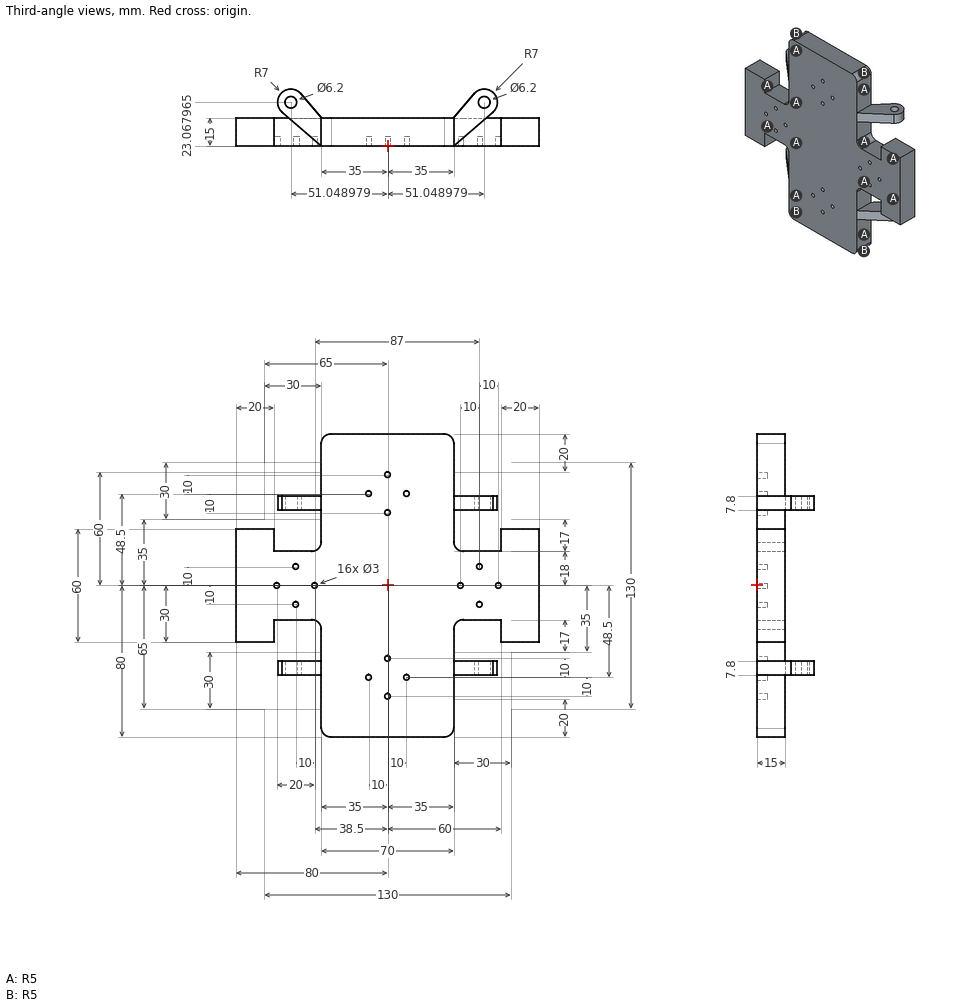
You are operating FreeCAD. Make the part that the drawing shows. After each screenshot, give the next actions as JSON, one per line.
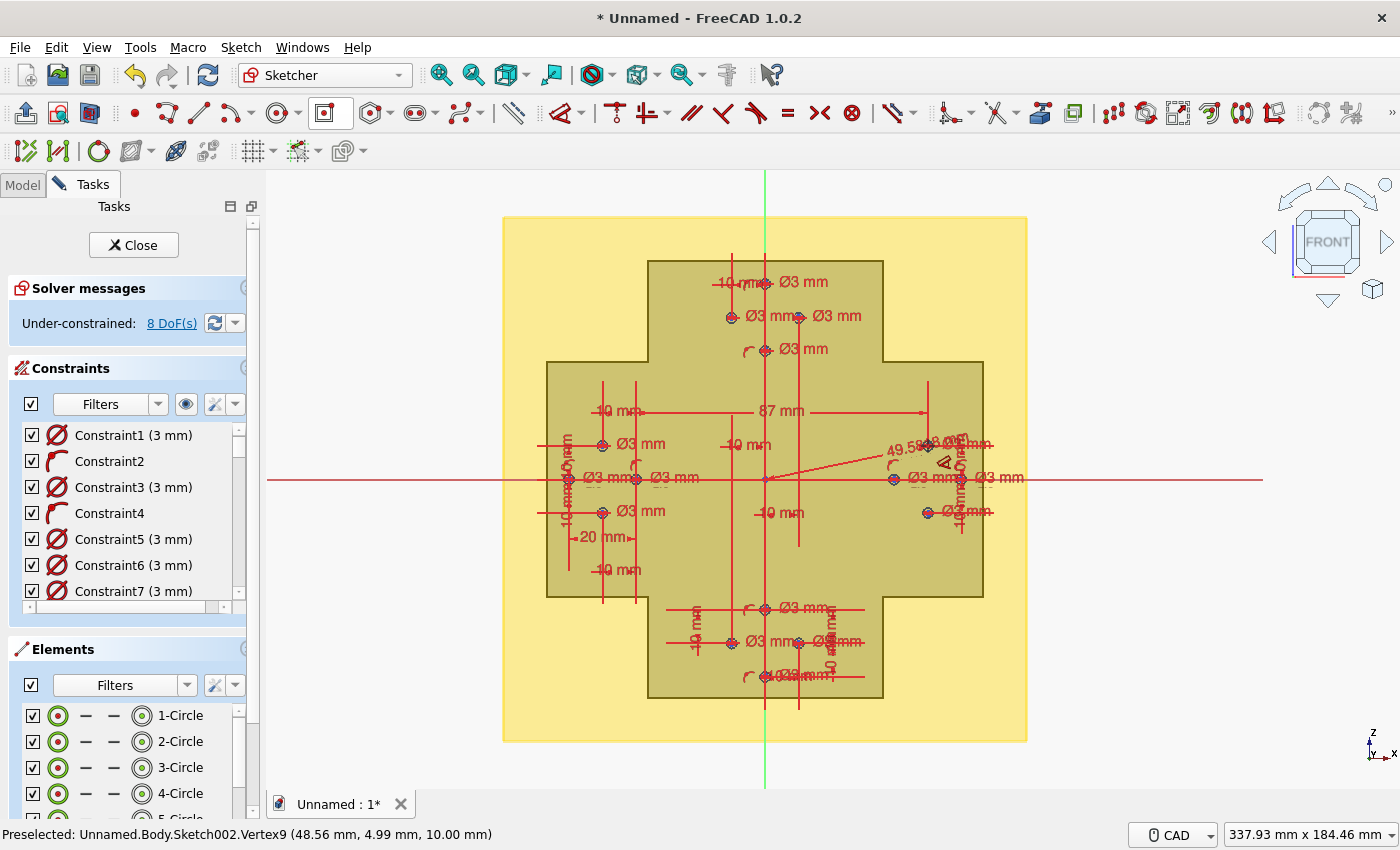
{"action": "left_click", "coordinate": [894, 480]}
{"action": "left_click", "coordinate": [911, 412]}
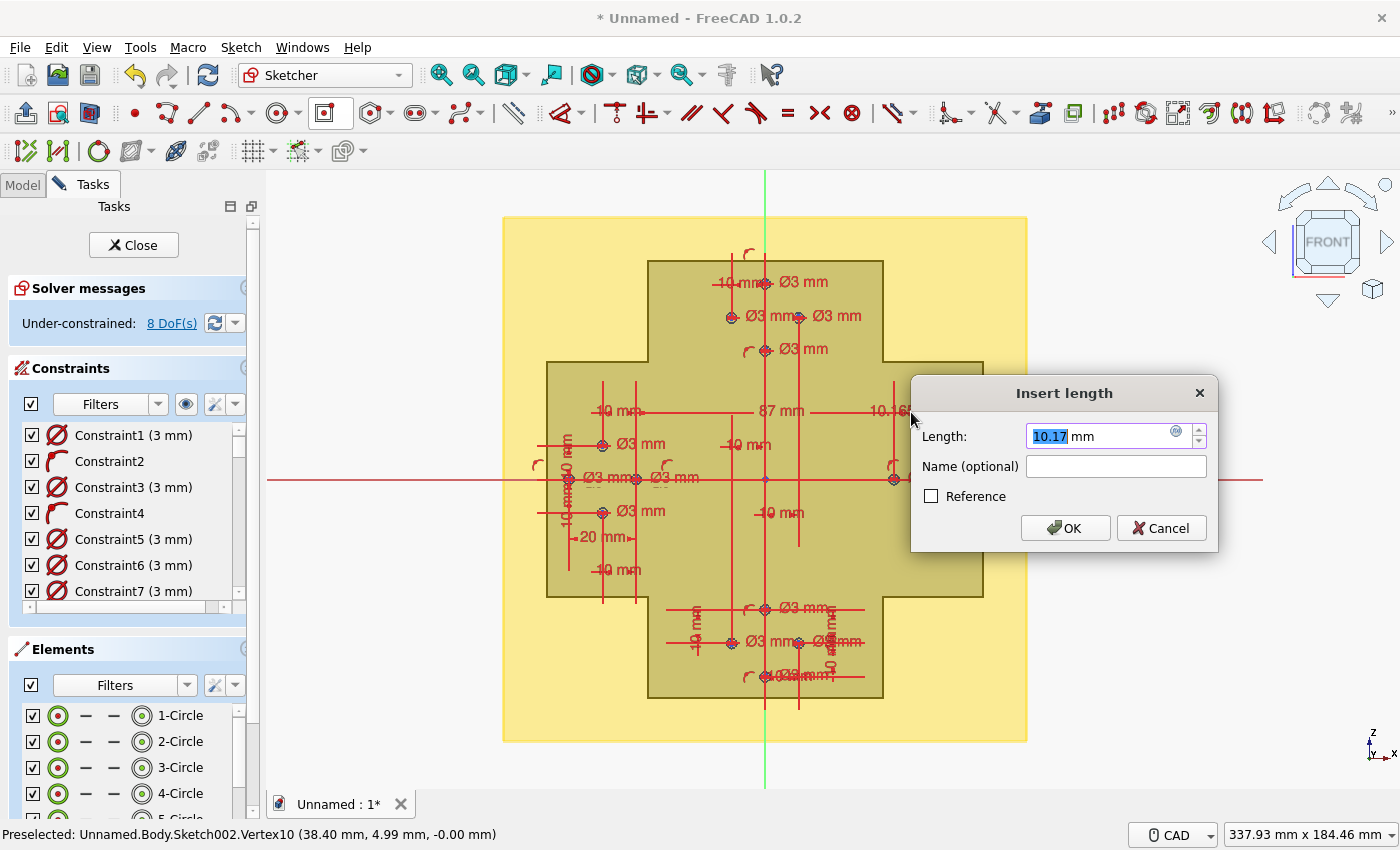
{"action": "type", "text": "10"}
{"action": "key", "text": "Return"}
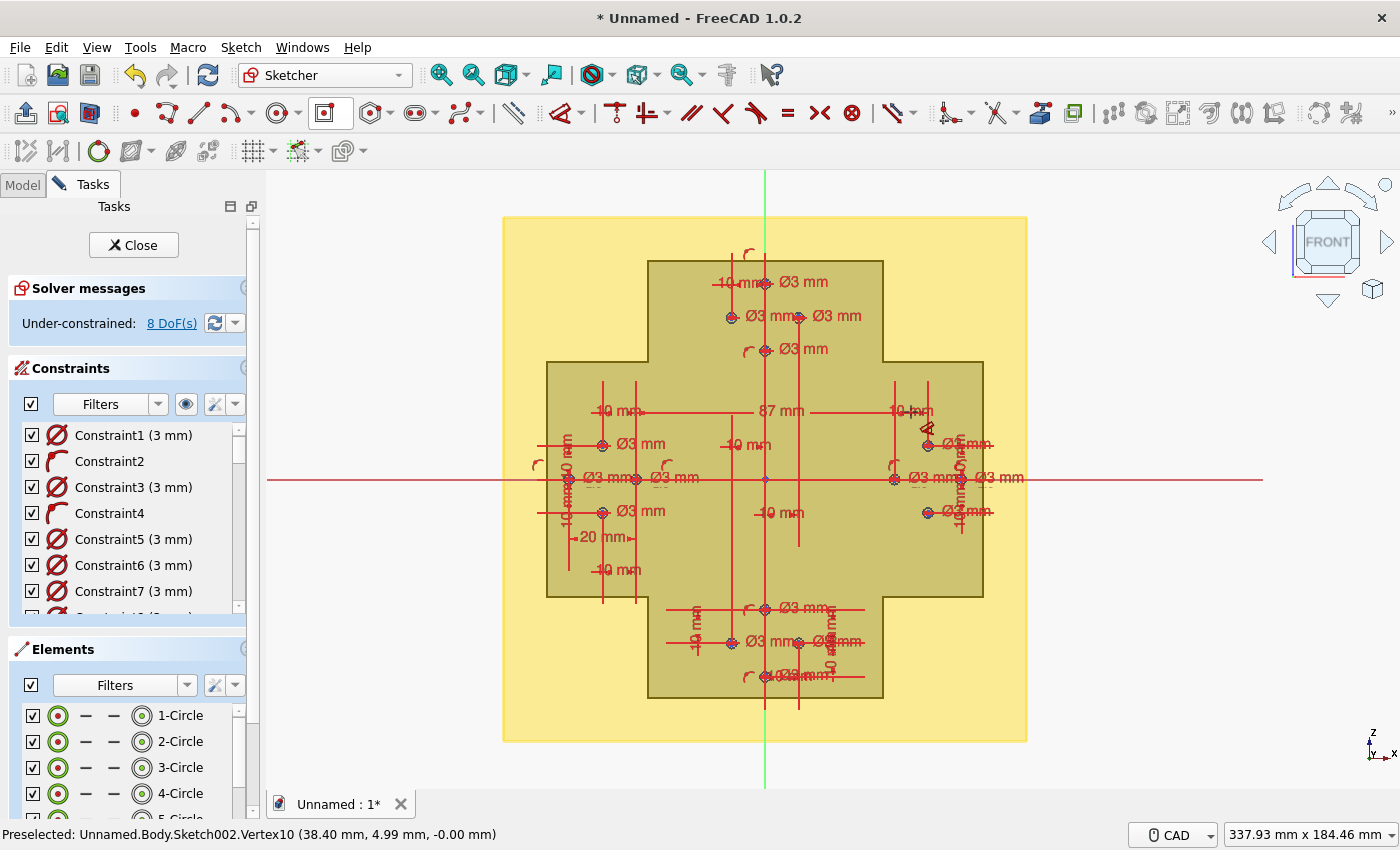
{"action": "left_click", "coordinate": [895, 480]}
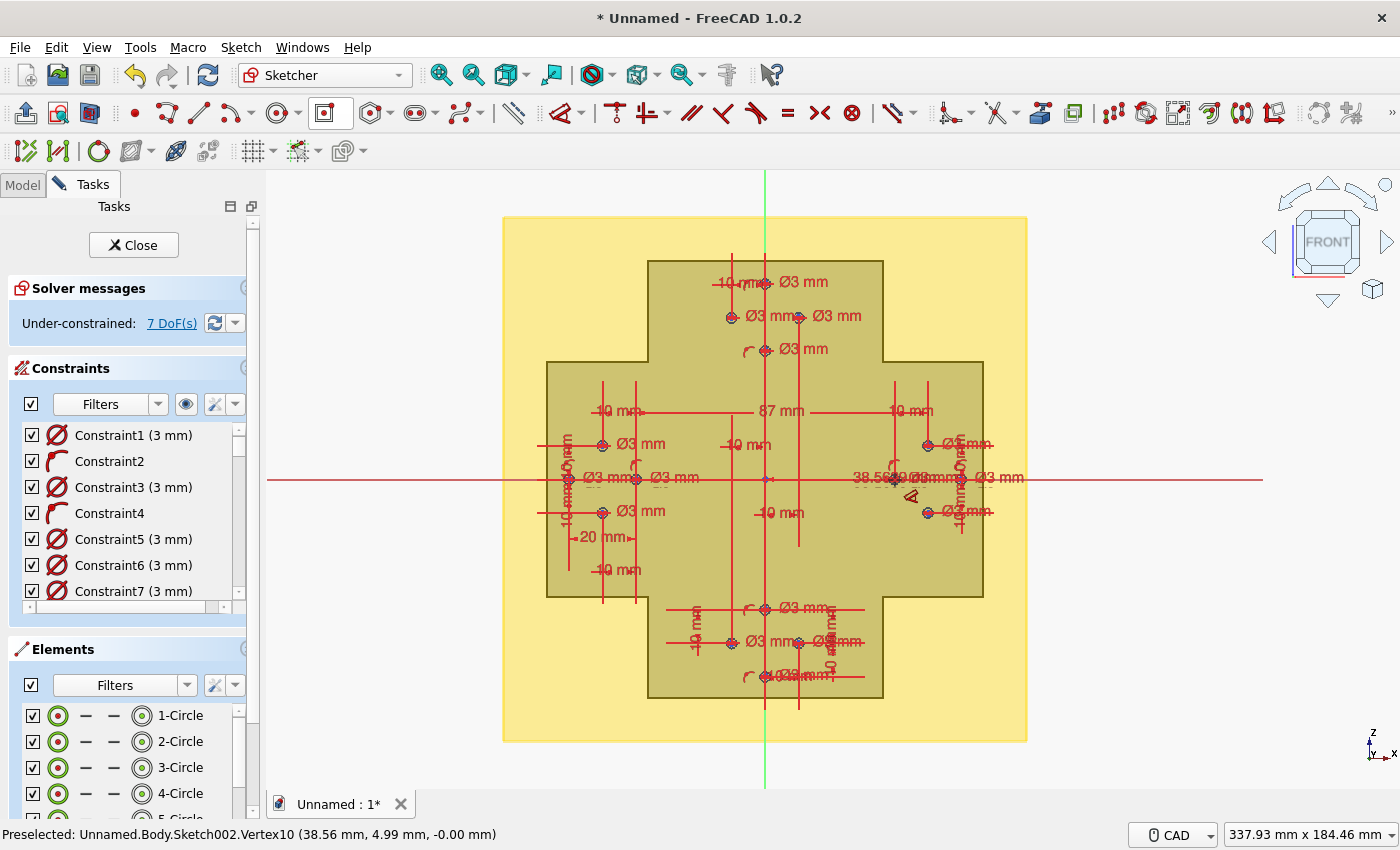
{"action": "left_click", "coordinate": [928, 513]}
{"action": "left_click", "coordinate": [911, 547]}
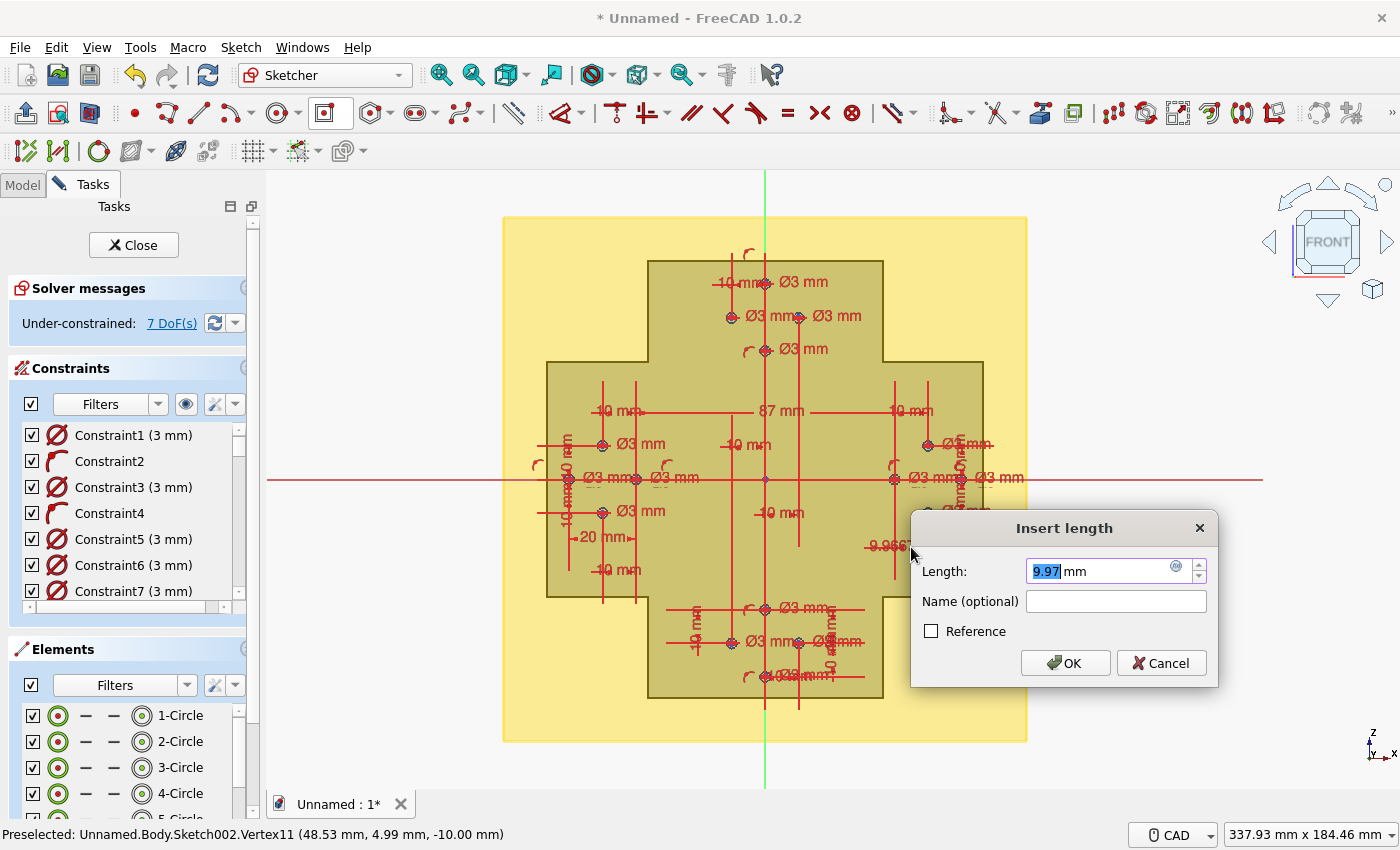
{"action": "type", "text": "10"}
{"action": "key", "text": "Return"}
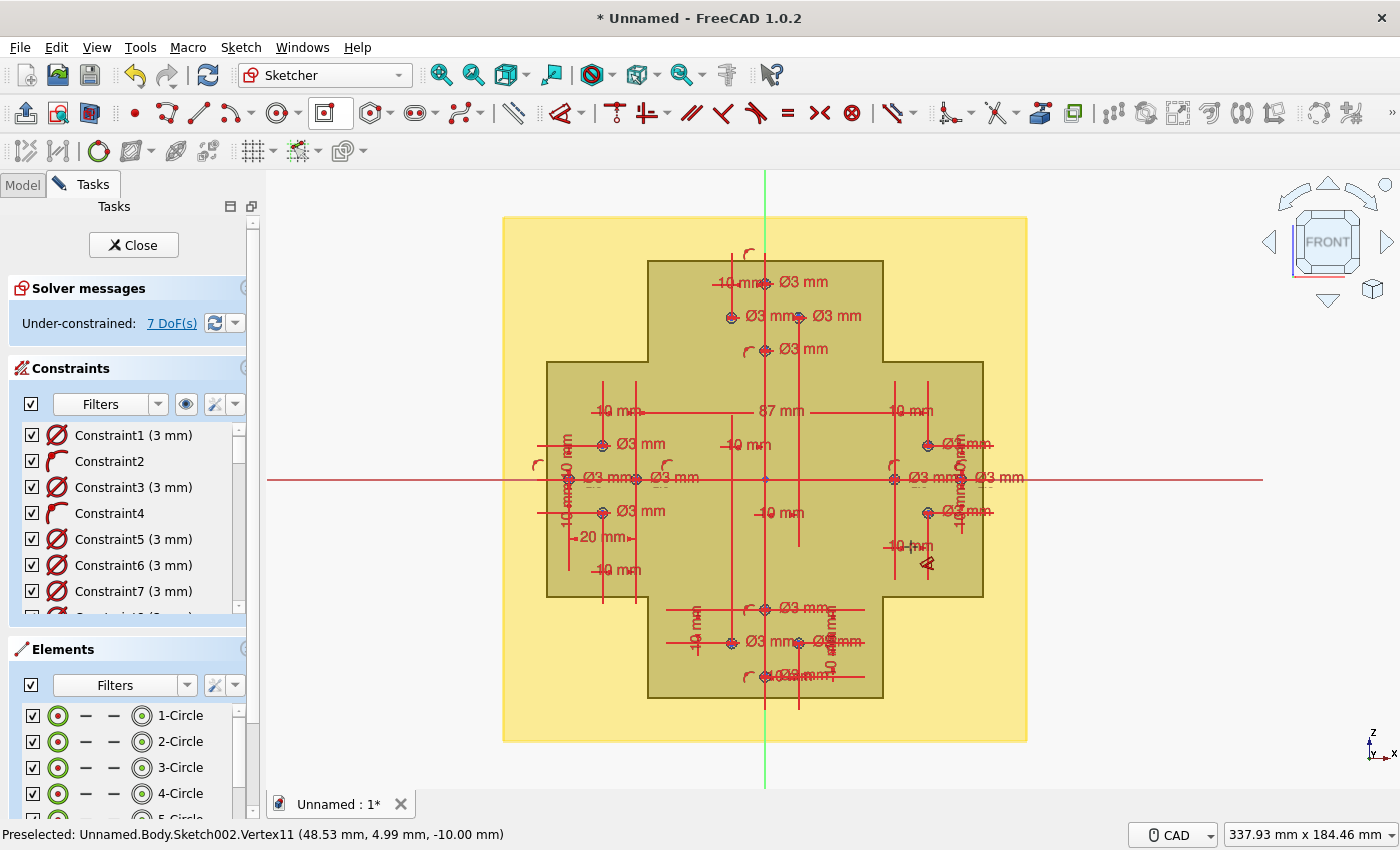
{"action": "left_click", "coordinate": [928, 446]}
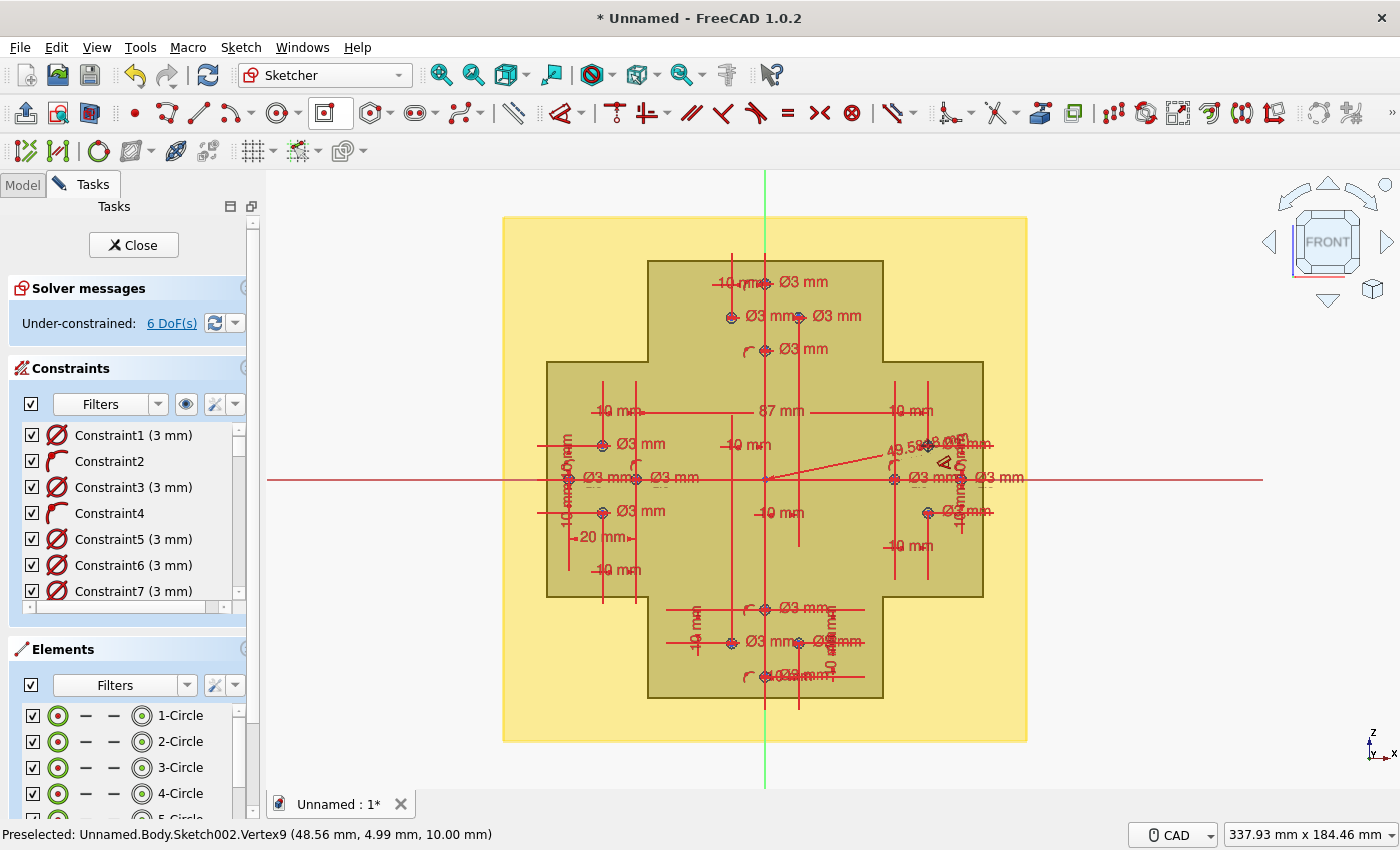
{"action": "left_click", "coordinate": [961, 480]}
{"action": "left_click", "coordinate": [945, 388]}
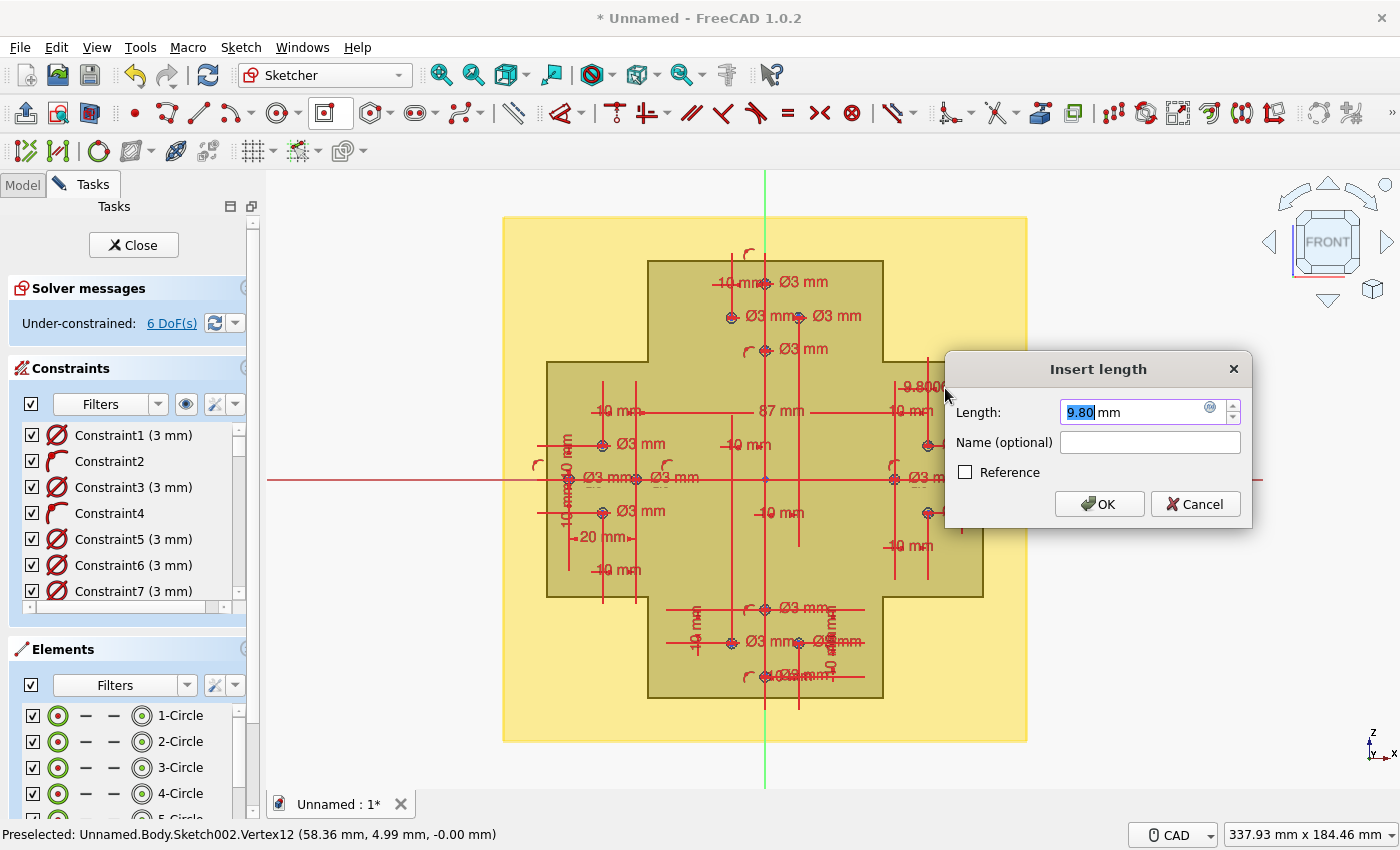
{"action": "type", "text": "10"}
{"action": "key", "text": "Return"}